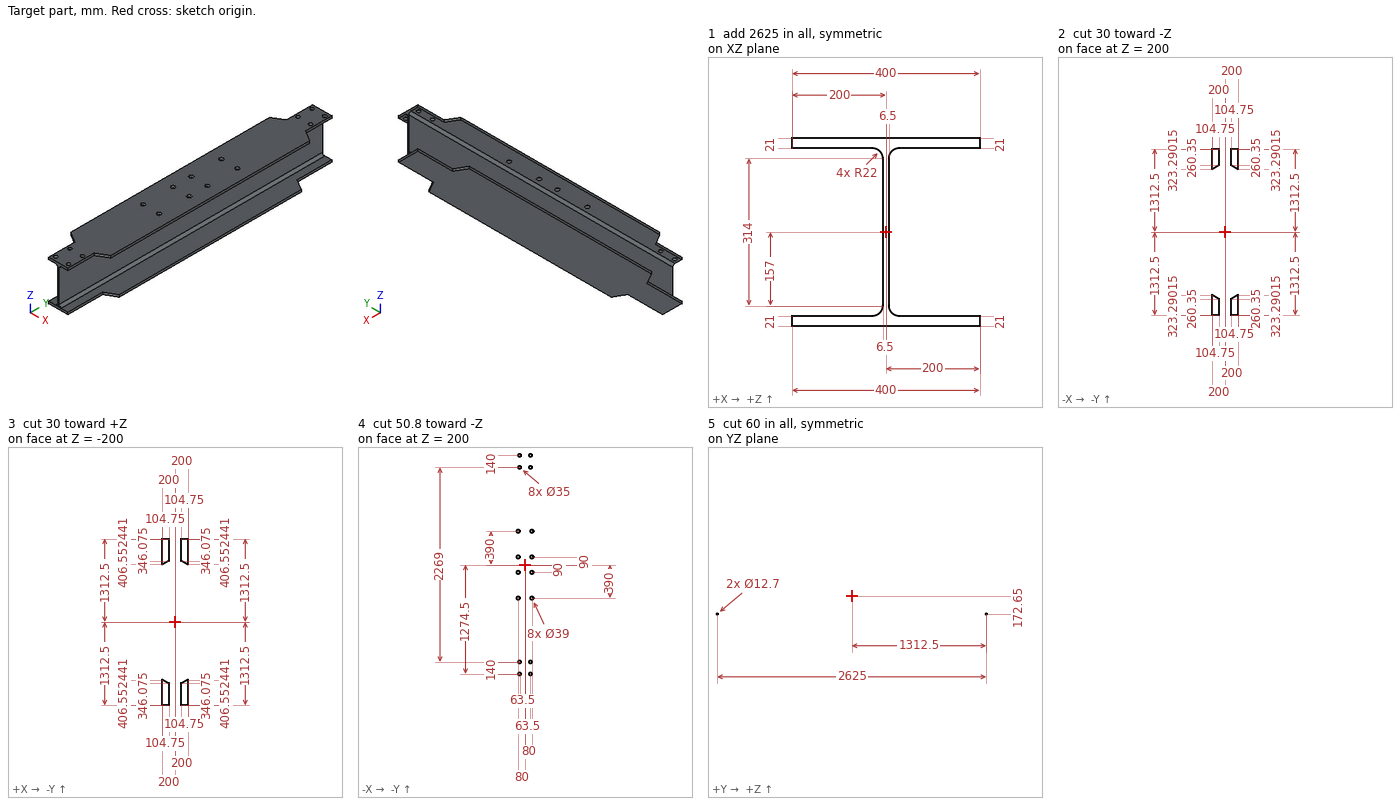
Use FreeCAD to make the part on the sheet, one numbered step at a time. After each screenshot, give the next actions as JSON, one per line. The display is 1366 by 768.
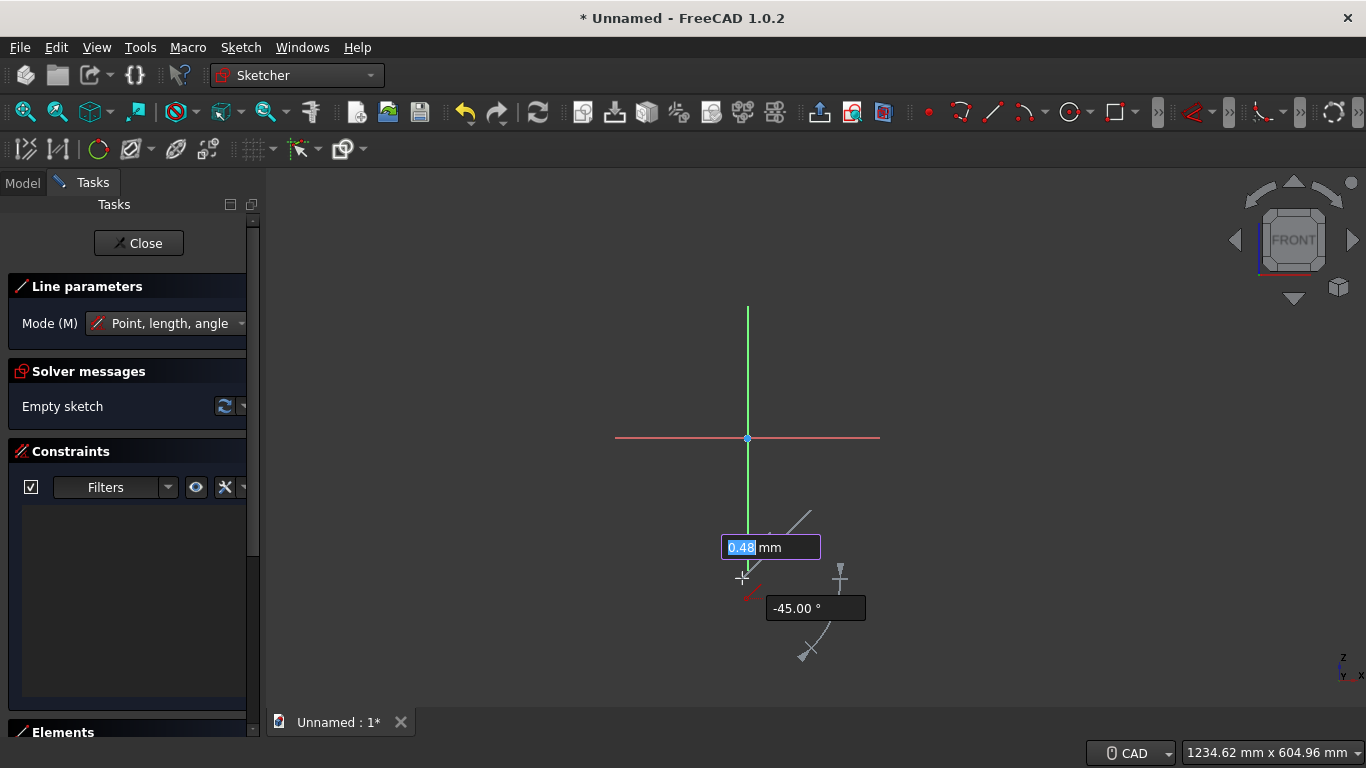
{"action": "scroll", "coordinate": [742, 298], "scroll_direction": "up", "scroll_amount": 6}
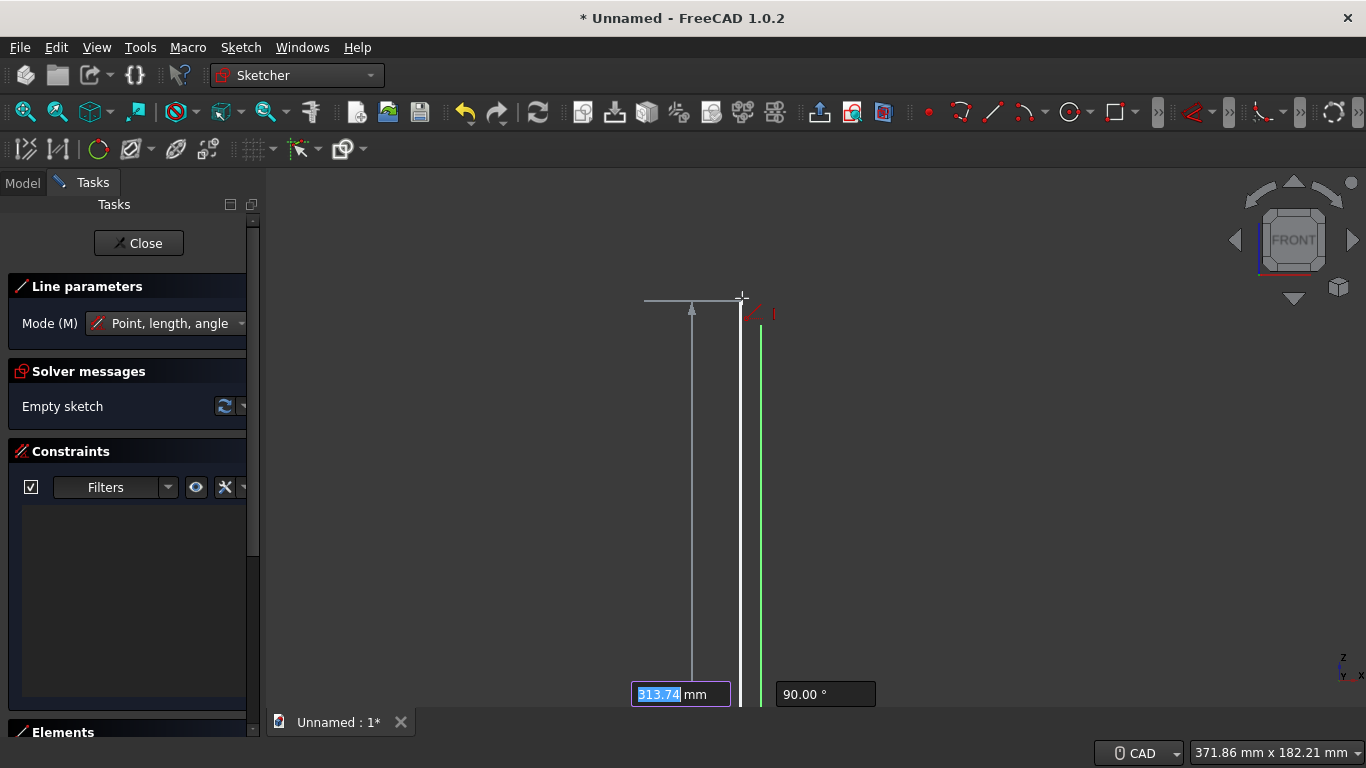
{"action": "left_click", "coordinate": [741, 299]}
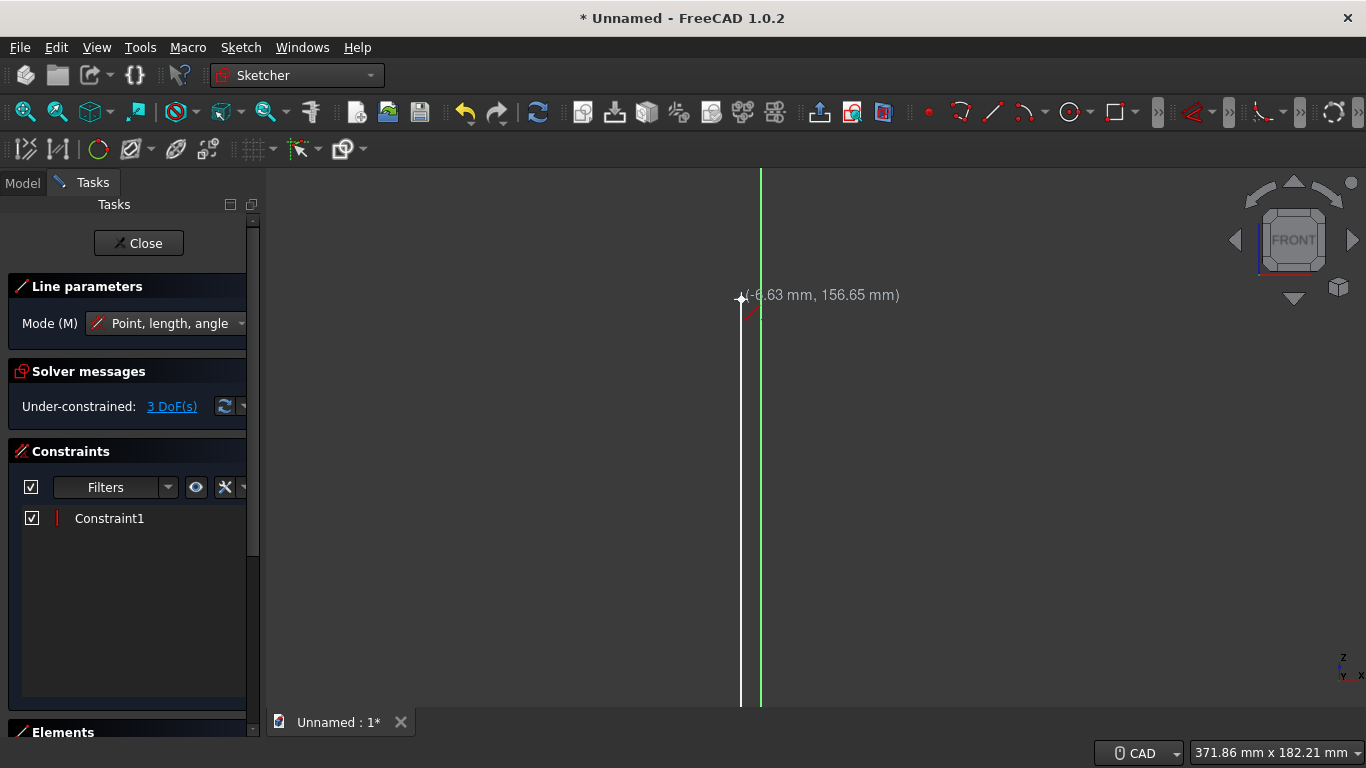
{"action": "left_click", "coordinate": [962, 112]}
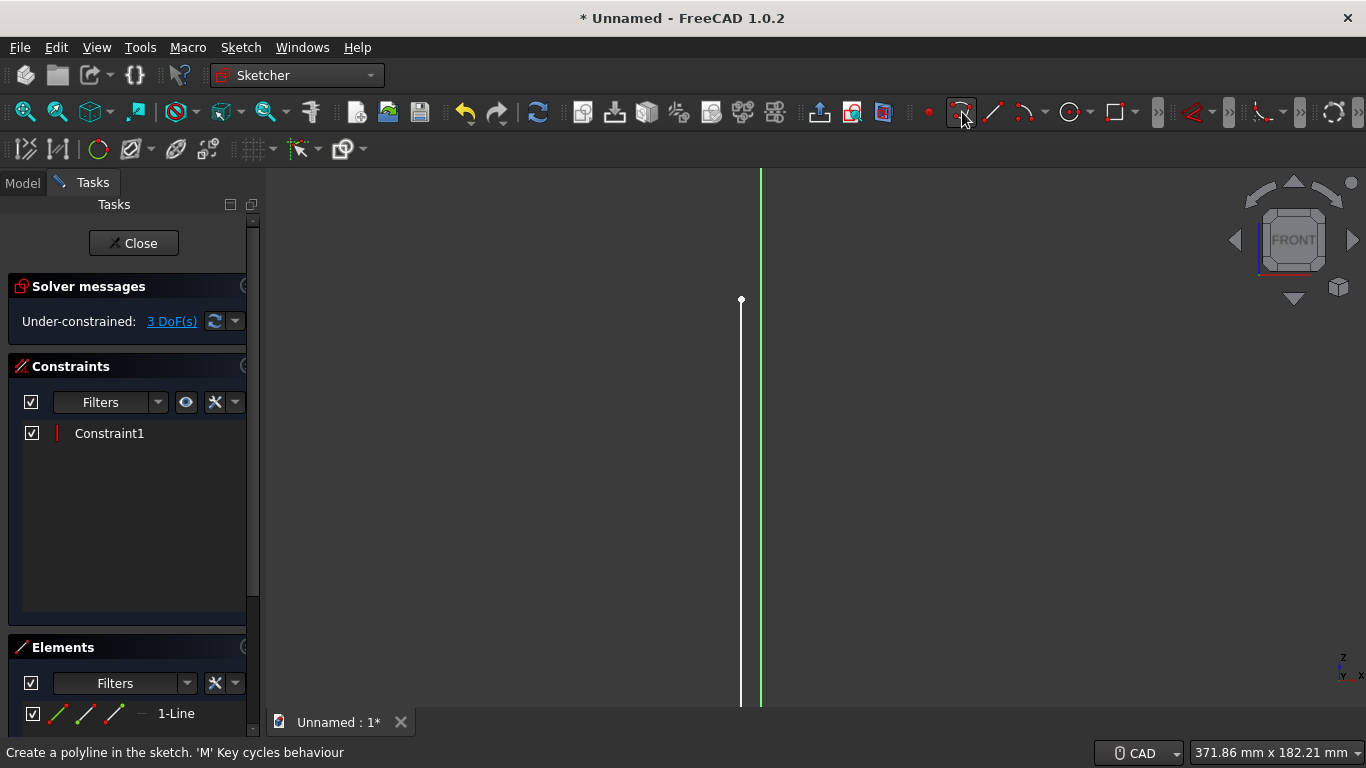
{"action": "left_click", "coordinate": [676, 234]}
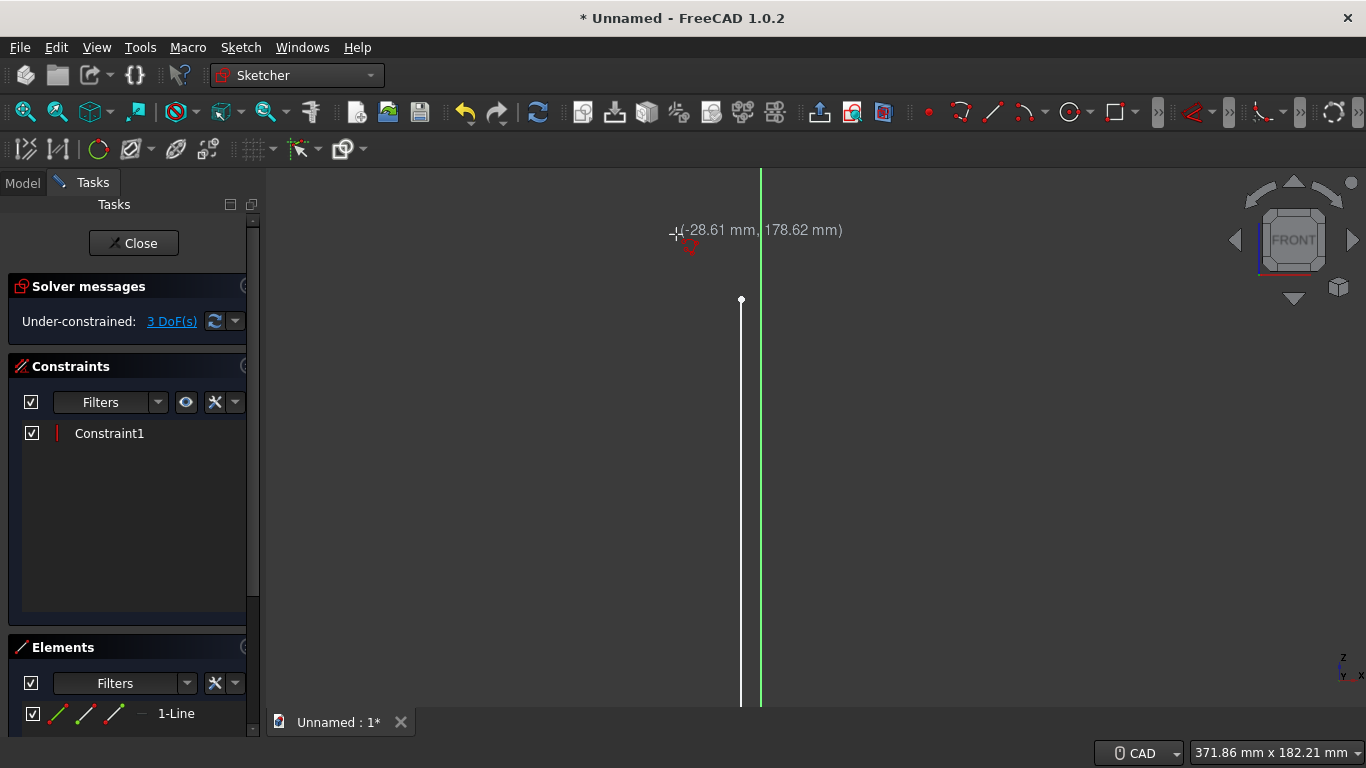
{"action": "scroll", "coordinate": [742, 297], "scroll_direction": "down", "scroll_amount": 6}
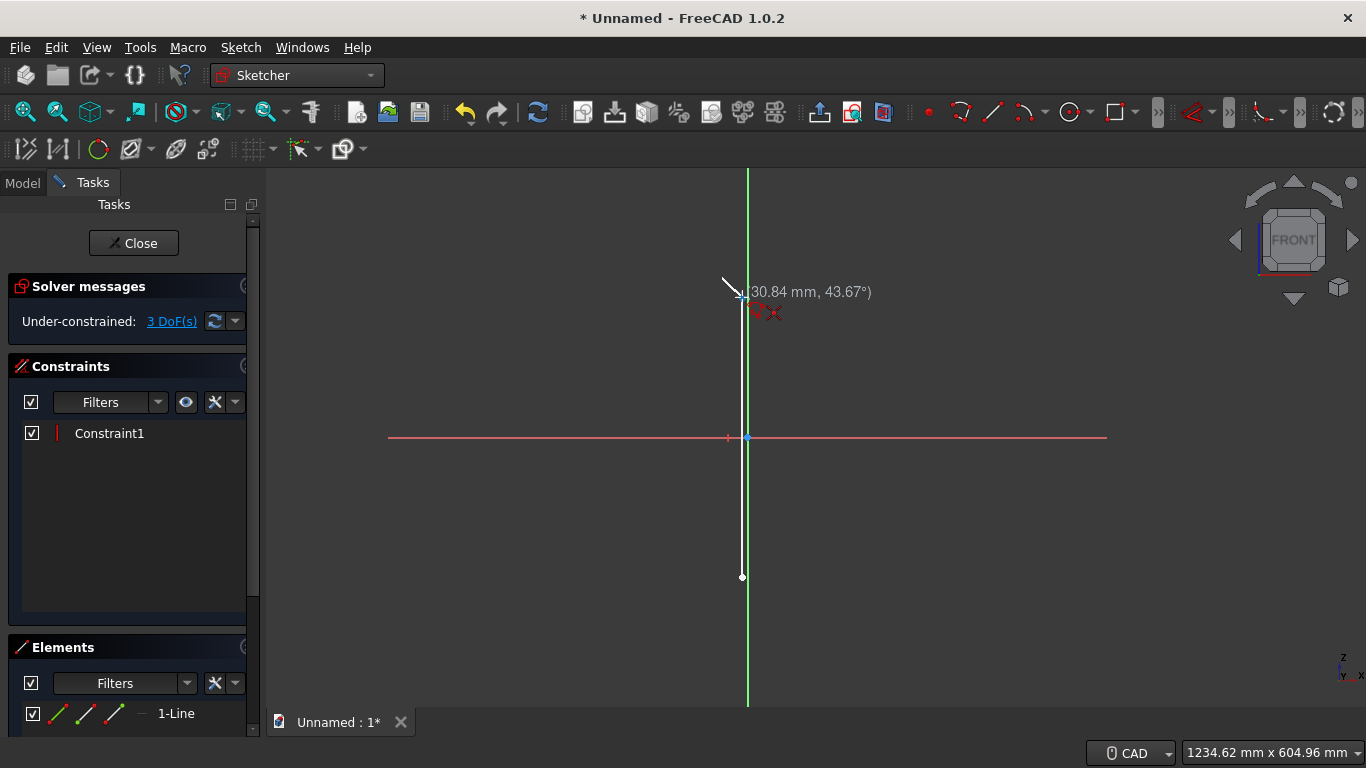
{"action": "left_click", "coordinate": [570, 278]}
{"action": "left_click", "coordinate": [570, 259]}
{"action": "left_click", "coordinate": [926, 259]}
{"action": "left_click", "coordinate": [926, 278]}
{"action": "left_click", "coordinate": [773, 278]}
{"action": "right_click", "coordinate": [773, 278]}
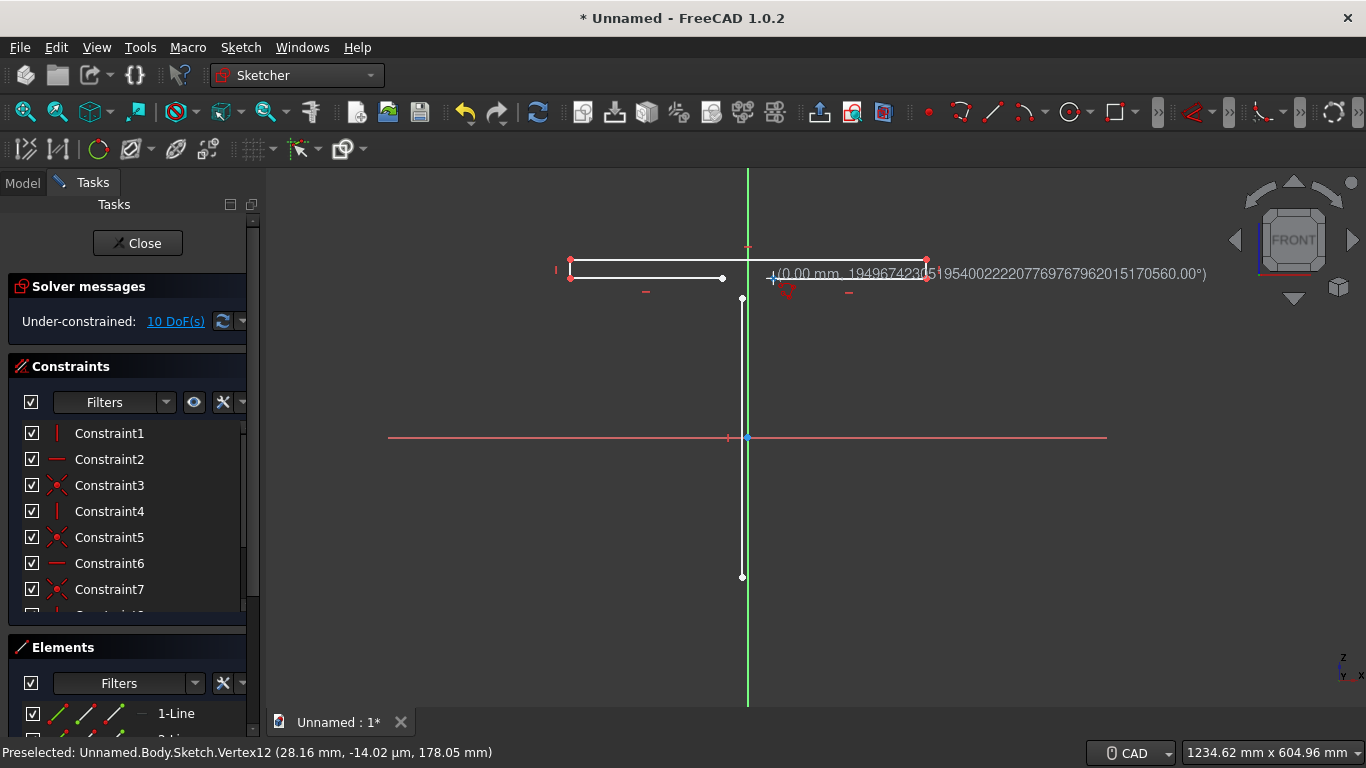
{"action": "left_click", "coordinate": [994, 112]}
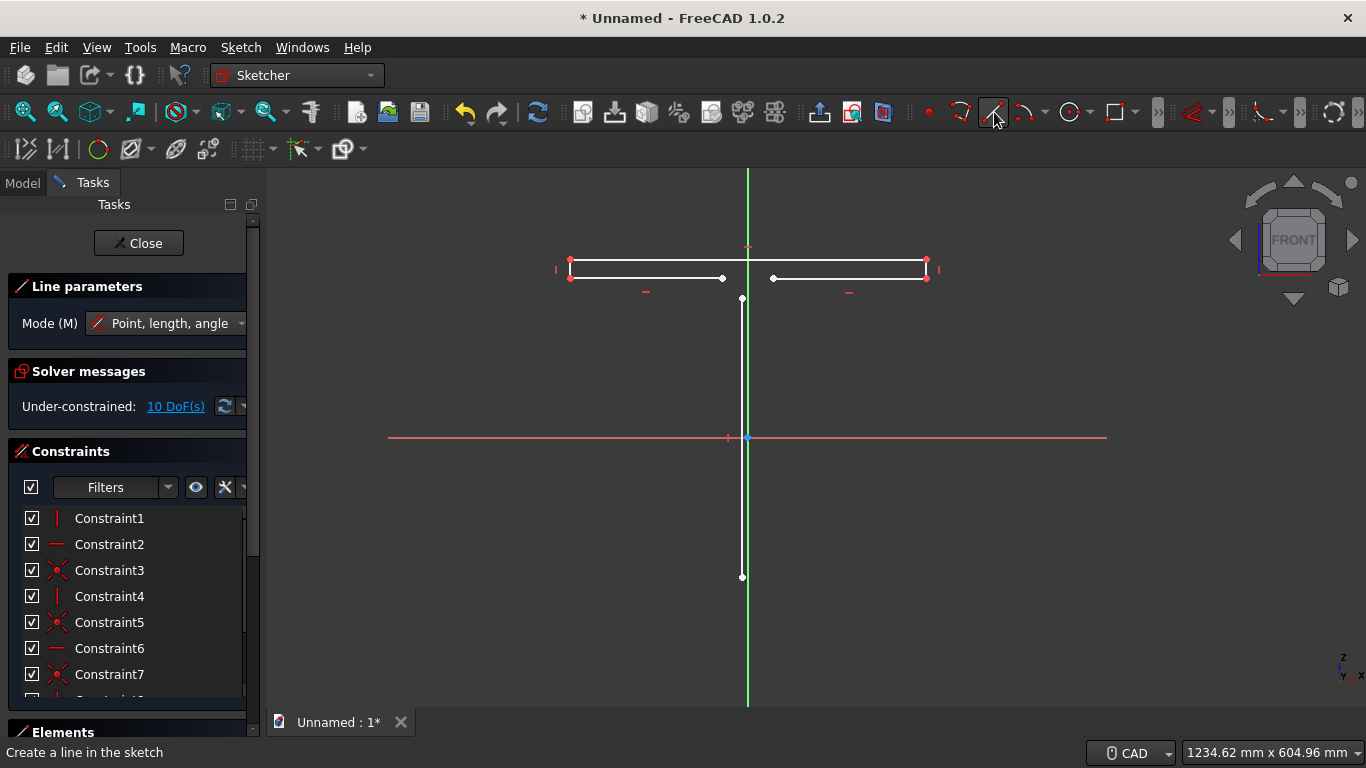
{"action": "scroll", "coordinate": [754, 298], "scroll_direction": "up", "scroll_amount": 6}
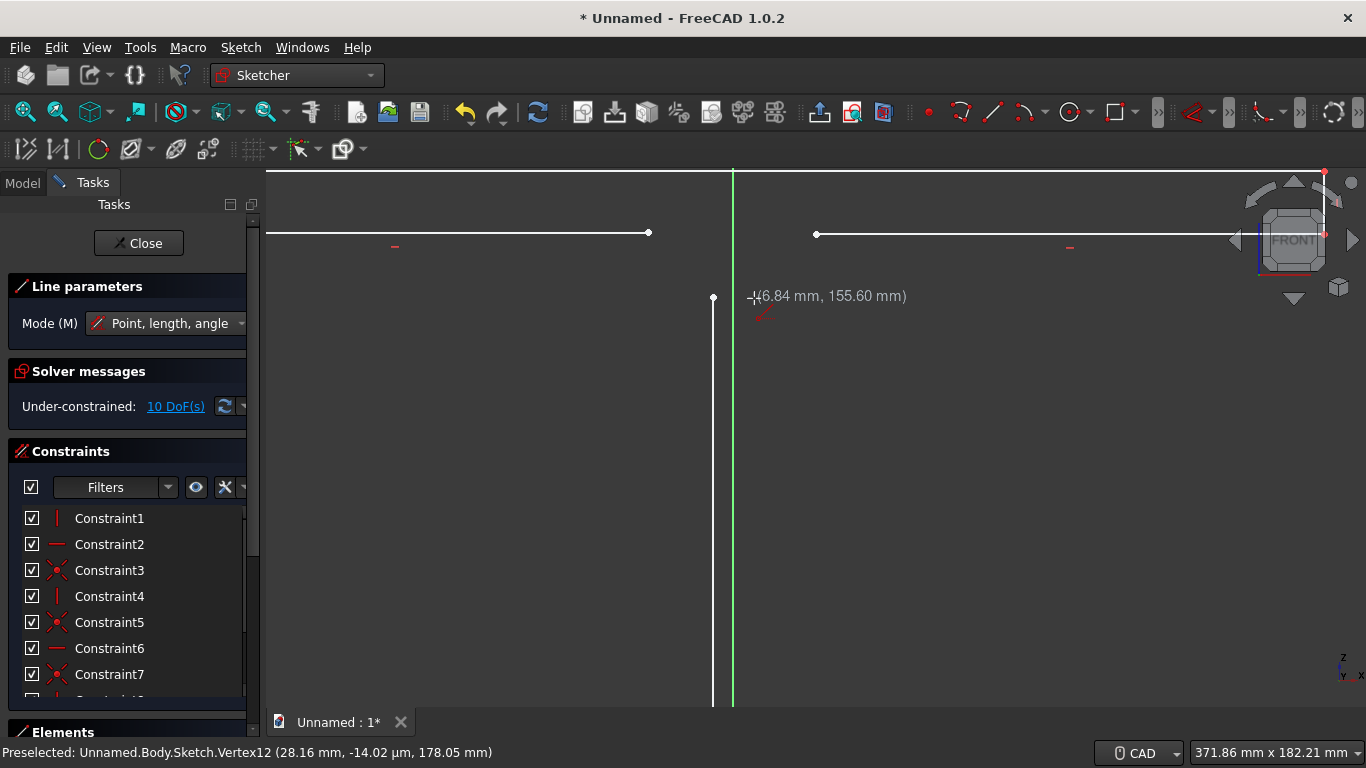
{"action": "left_click", "coordinate": [752, 297]}